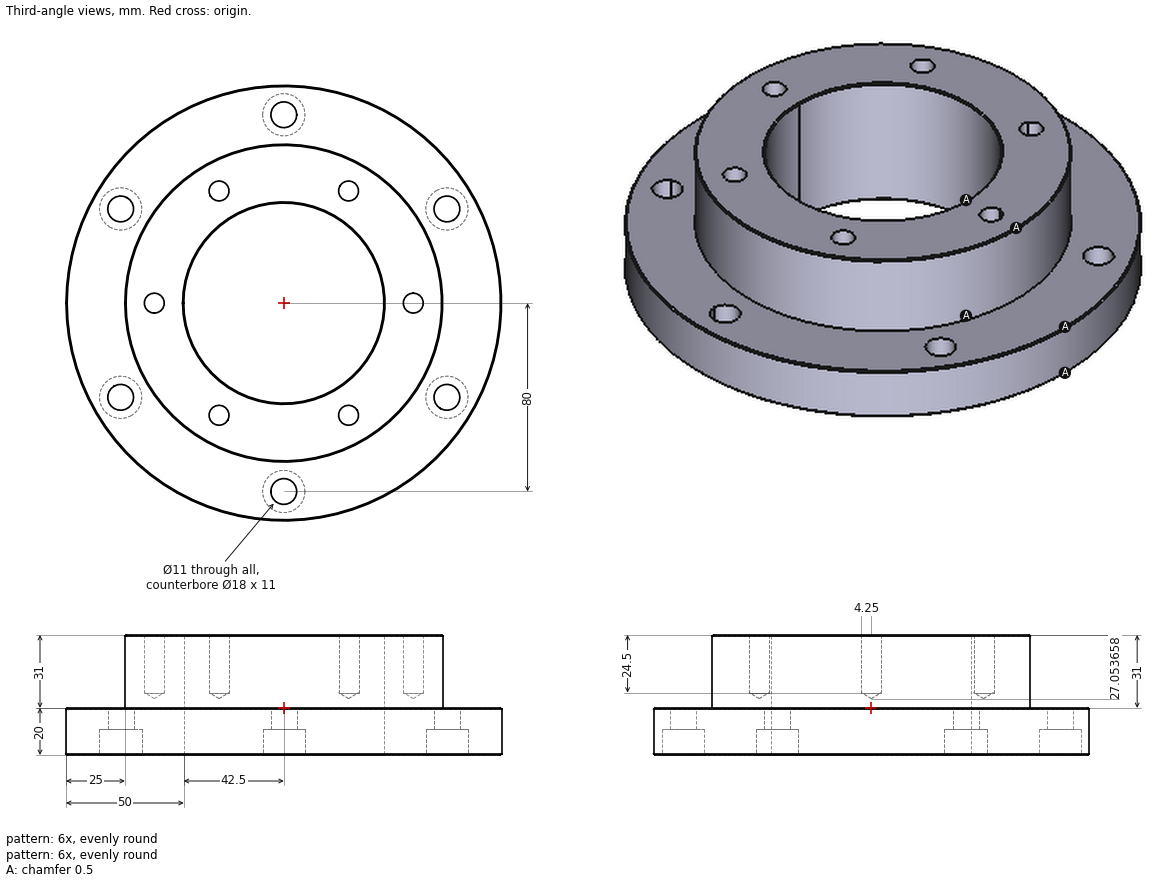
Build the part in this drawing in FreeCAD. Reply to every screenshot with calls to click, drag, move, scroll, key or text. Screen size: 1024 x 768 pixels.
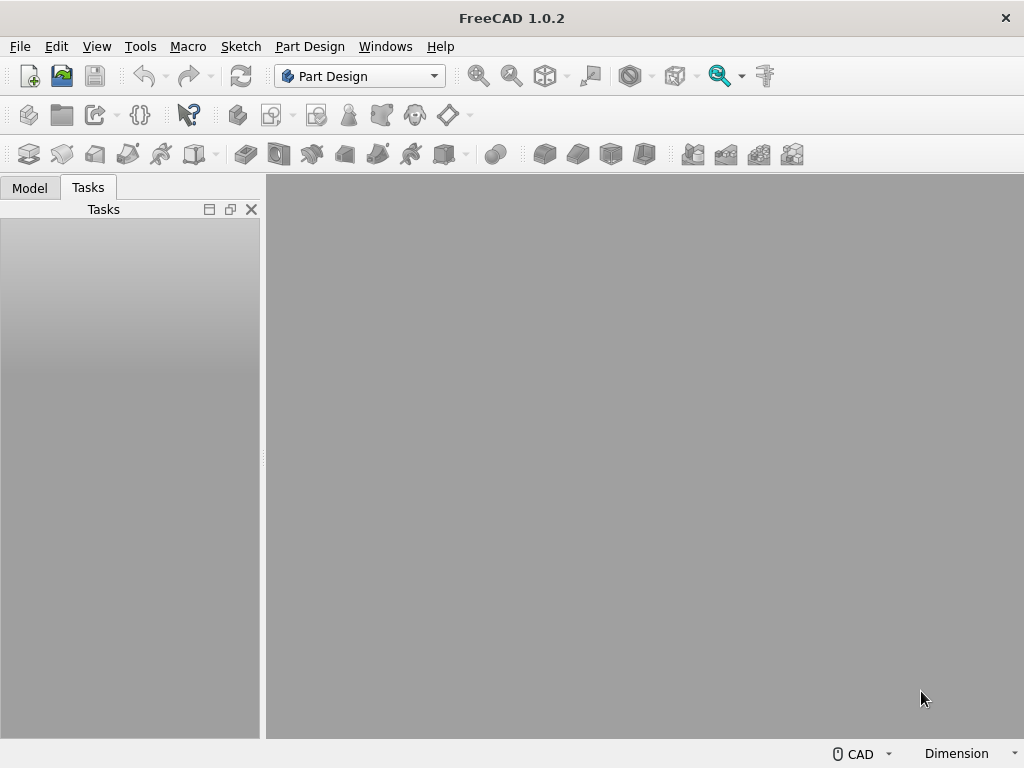
key(ctrl+n)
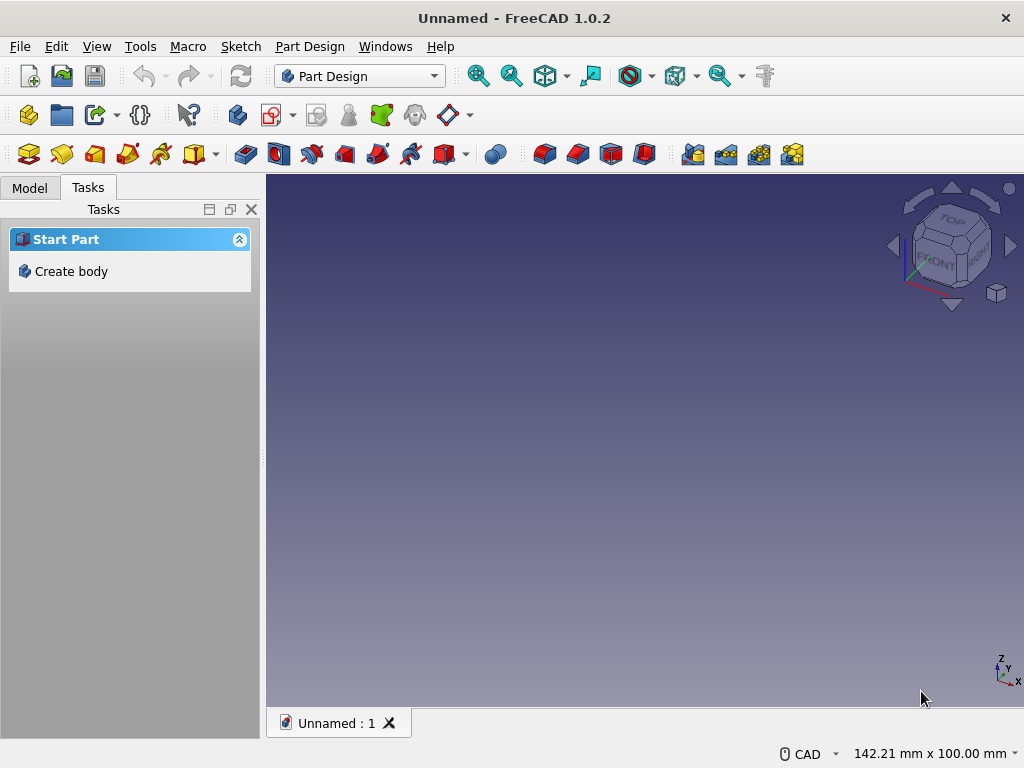
click(270, 116)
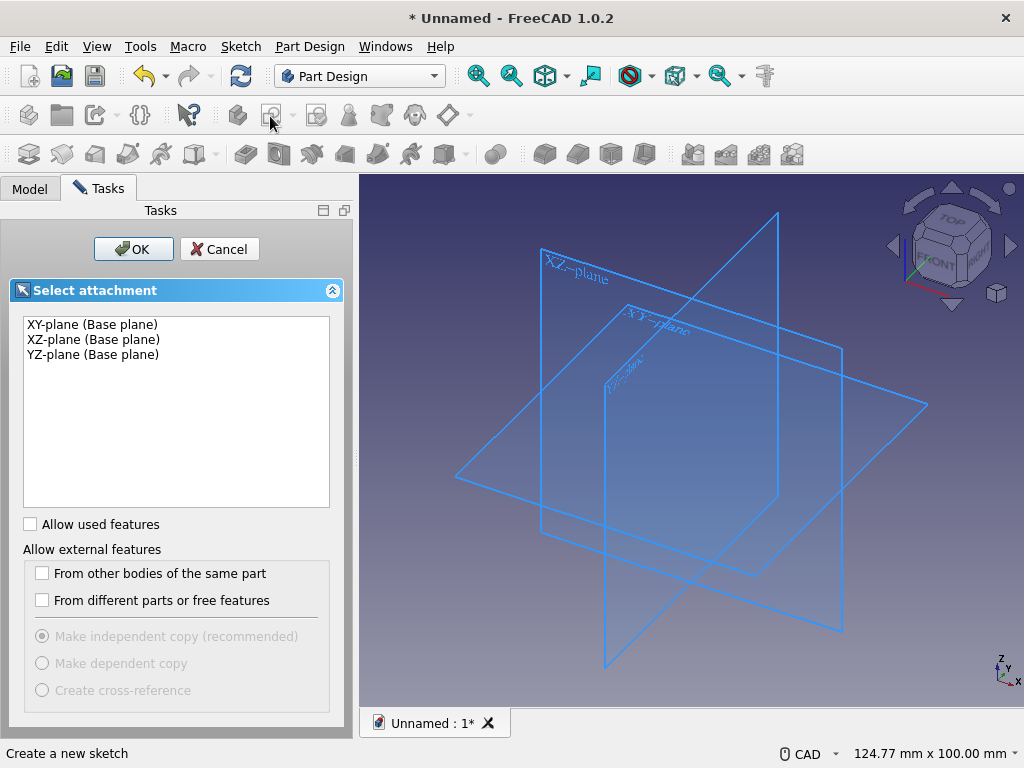
click(84, 340)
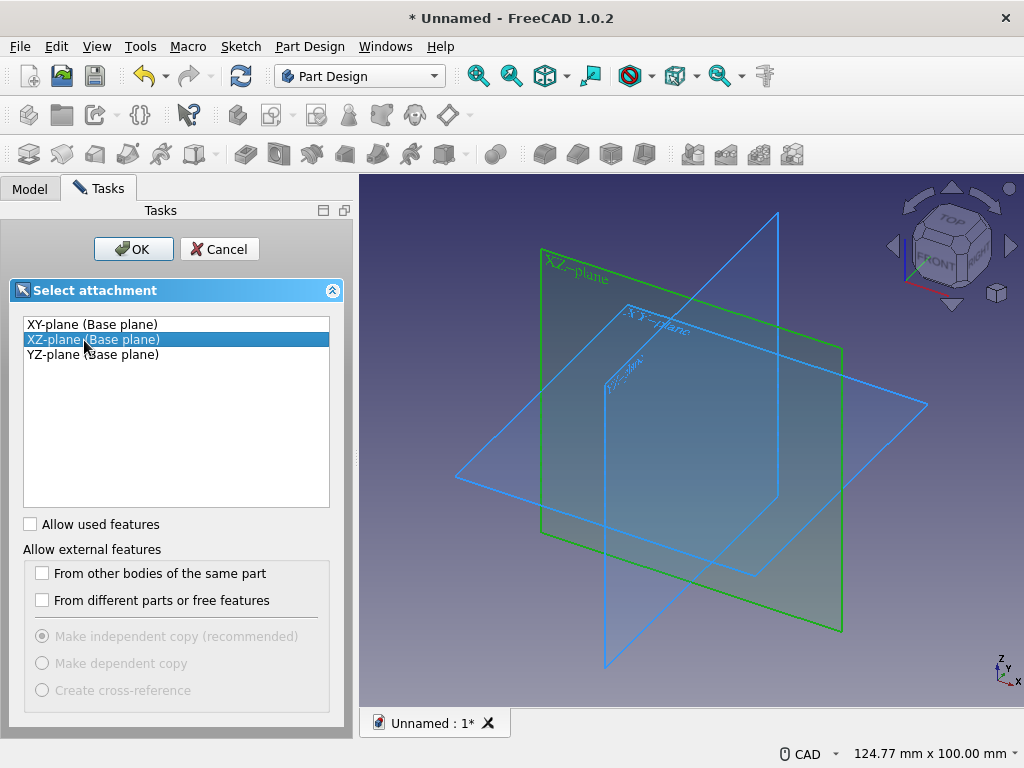
click(134, 249)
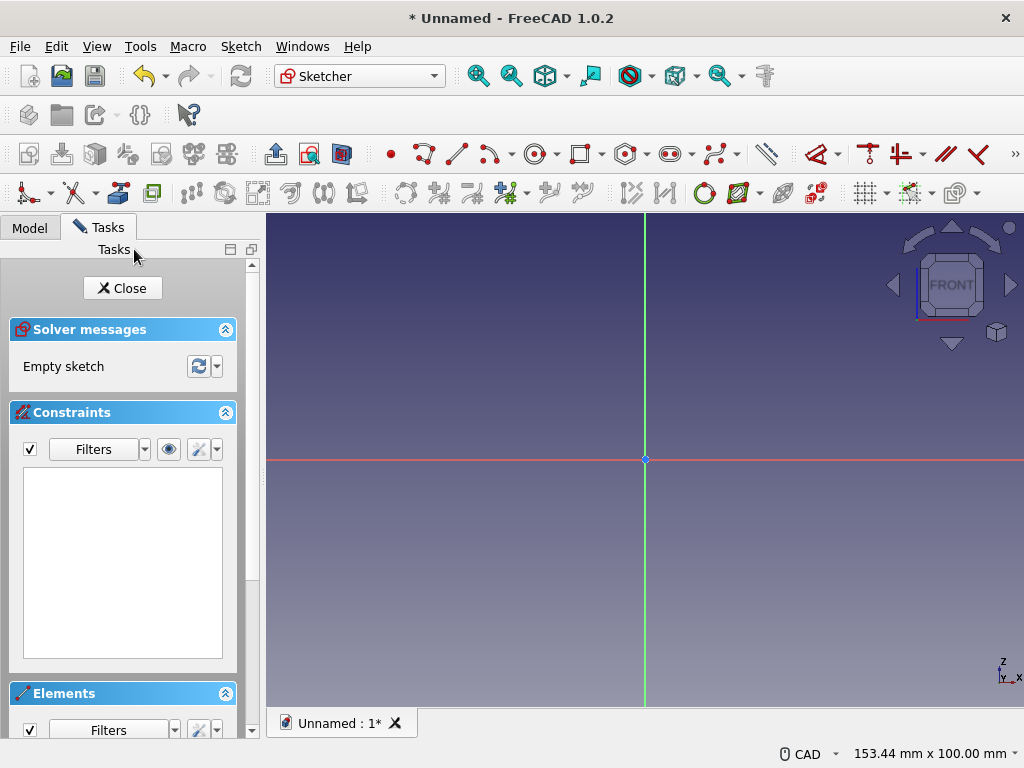
scroll(859, 515, down, 2)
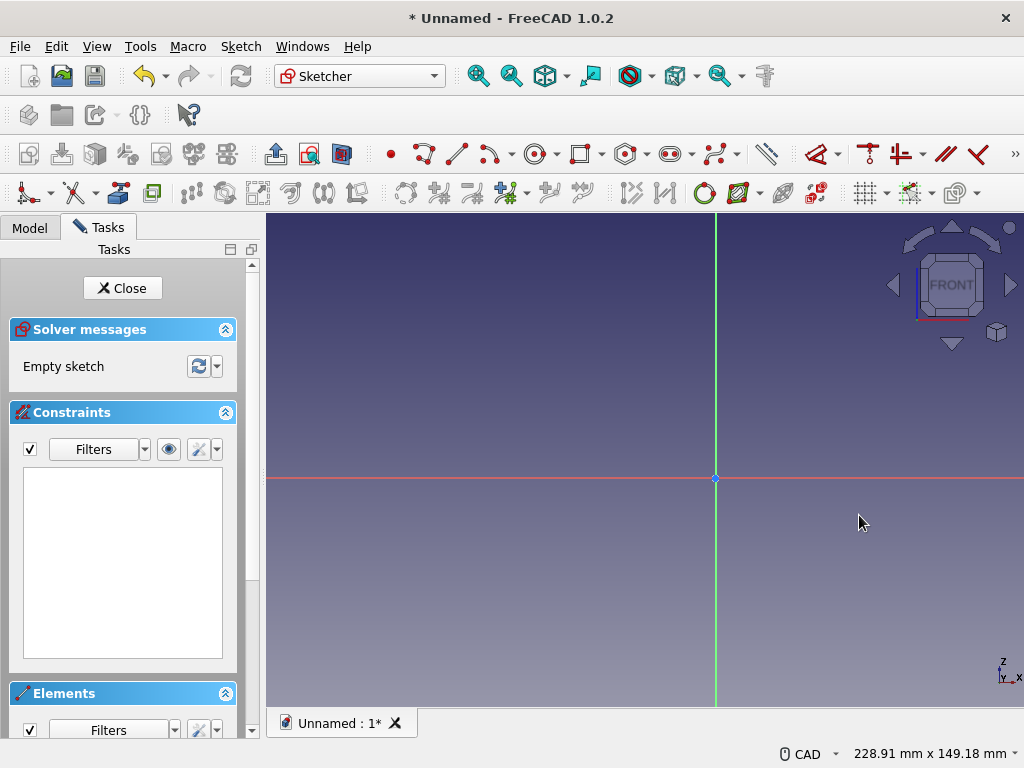
click(424, 154)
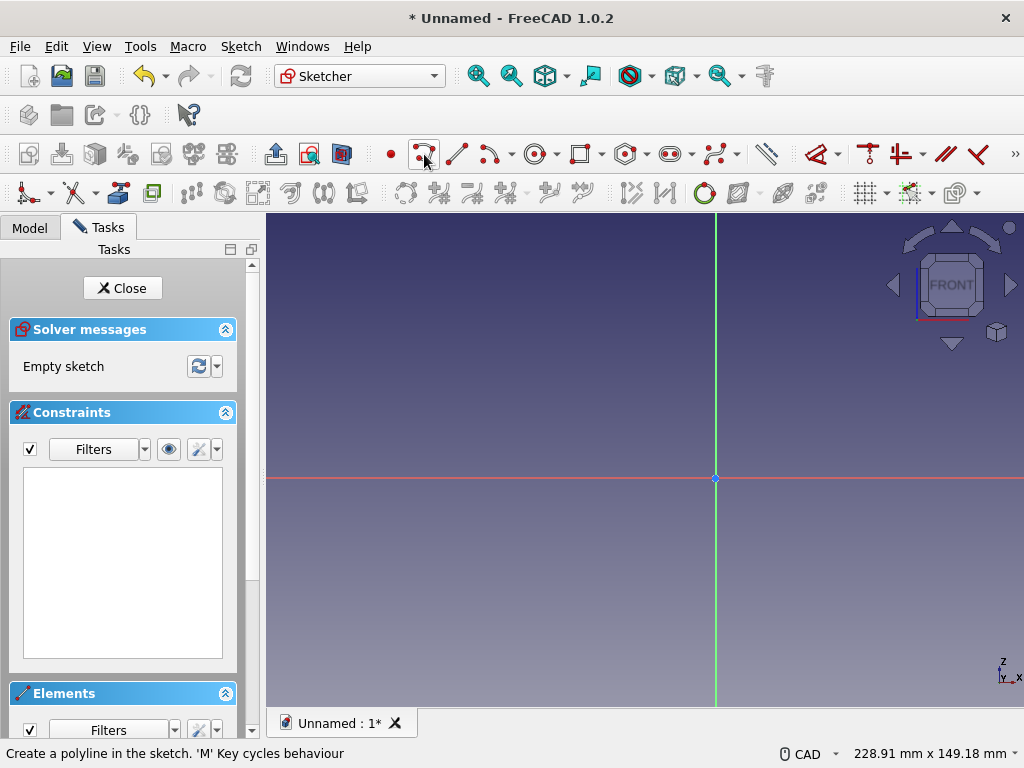
click(575, 545)
click(410, 545)
click(410, 478)
click(492, 469)
click(492, 376)
click(575, 376)
click(575, 546)
key(Escape)
key(Escape)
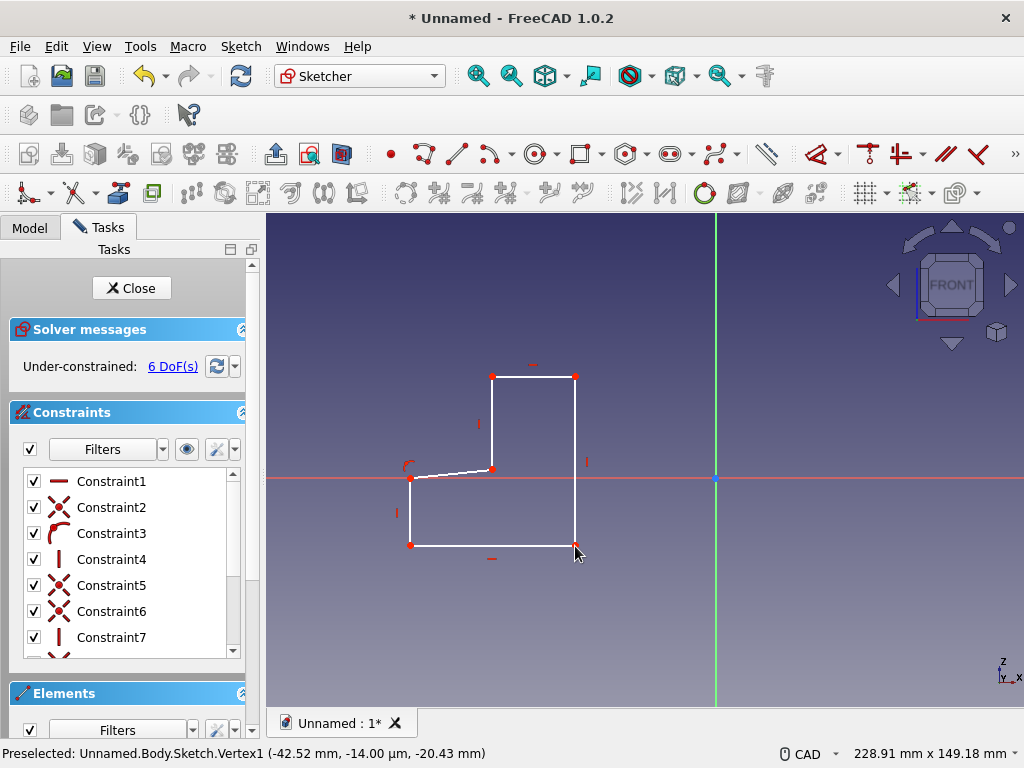
click(435, 476)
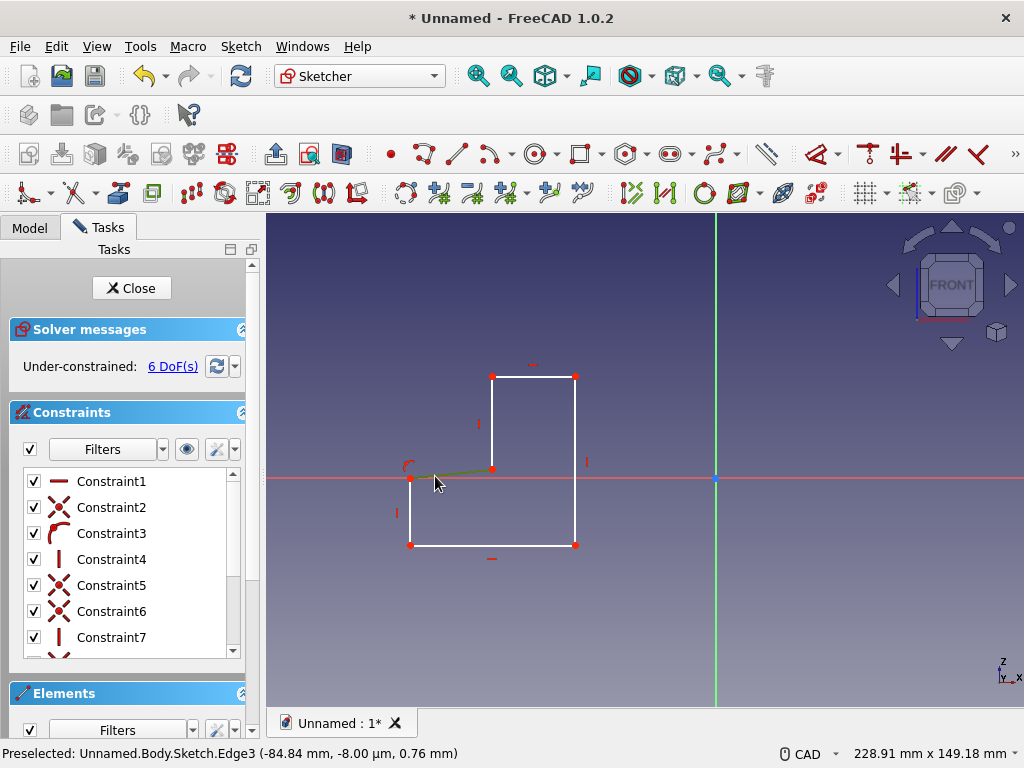
key(h)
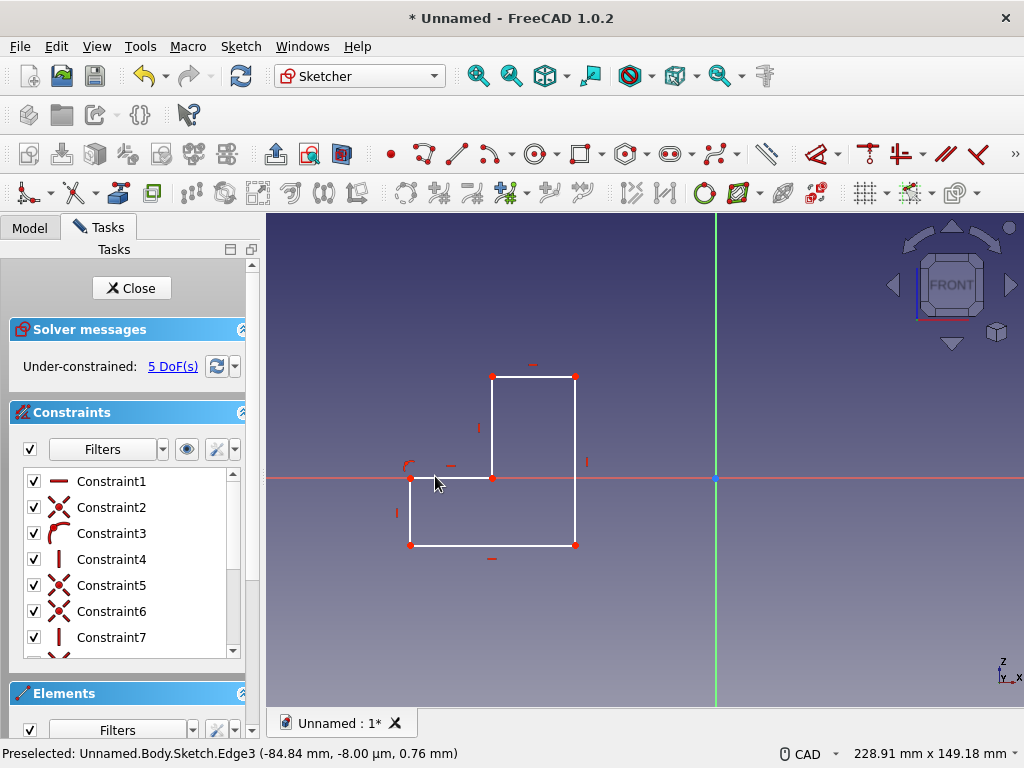
click(525, 546)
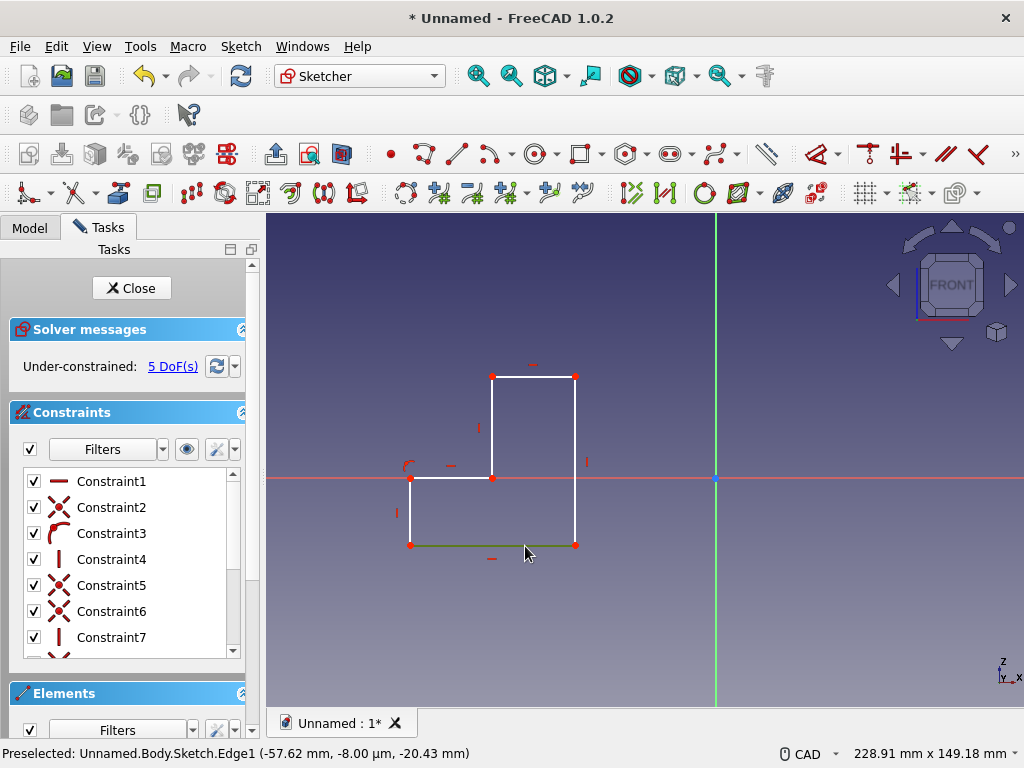
click(838, 154)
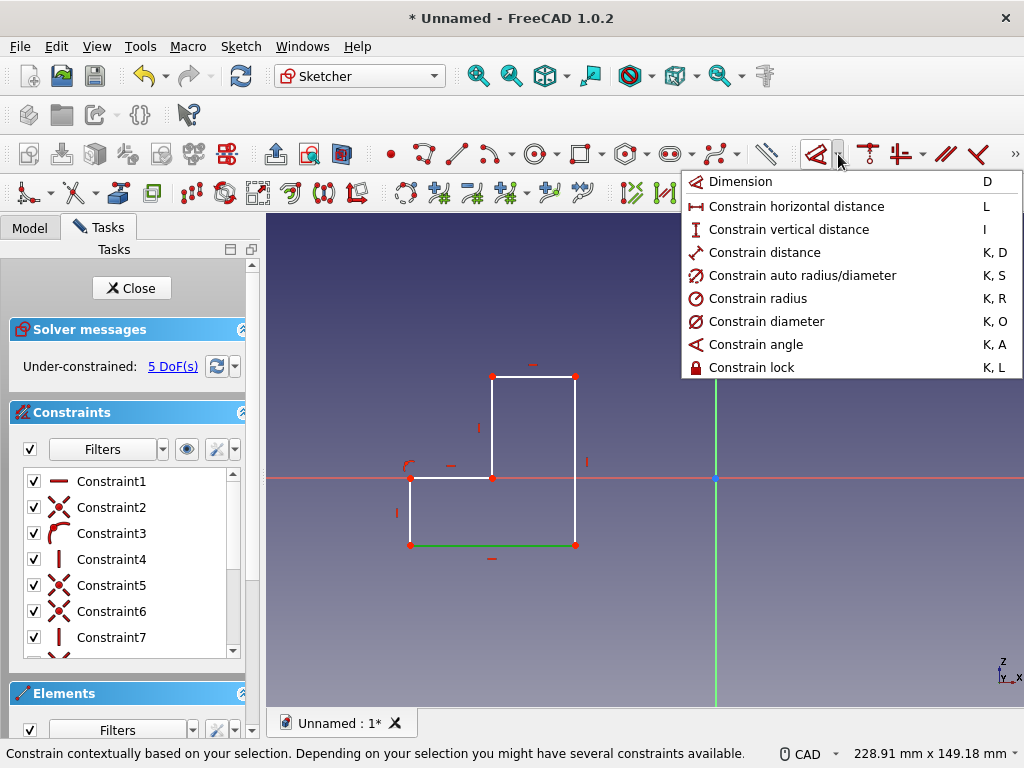
click(852, 206)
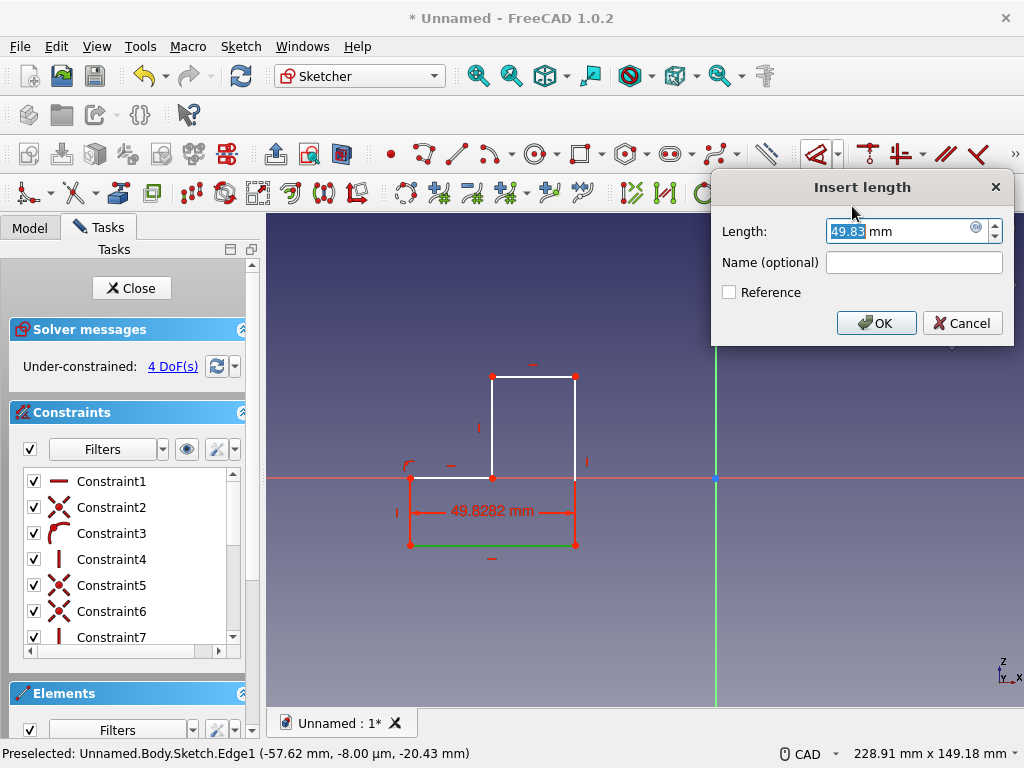
text(50)
key(Return)